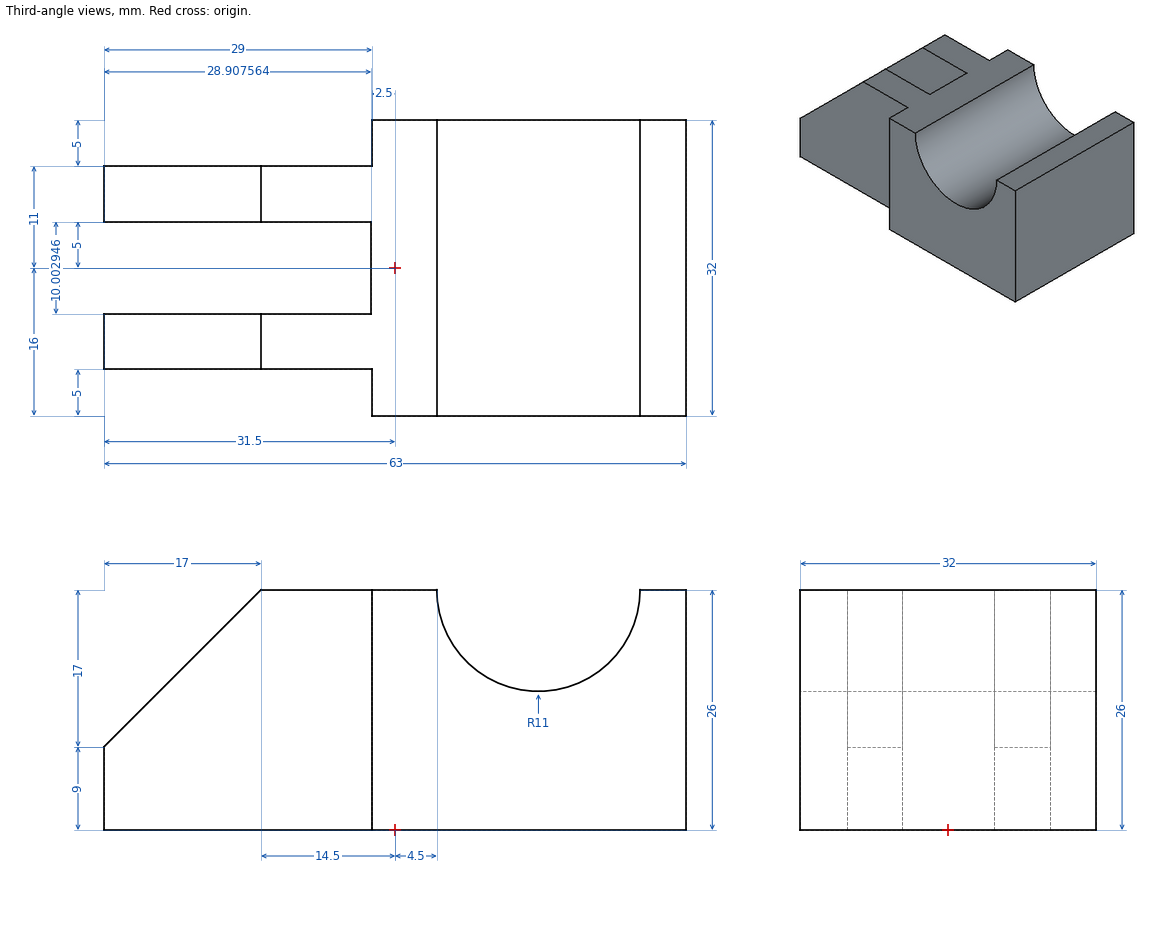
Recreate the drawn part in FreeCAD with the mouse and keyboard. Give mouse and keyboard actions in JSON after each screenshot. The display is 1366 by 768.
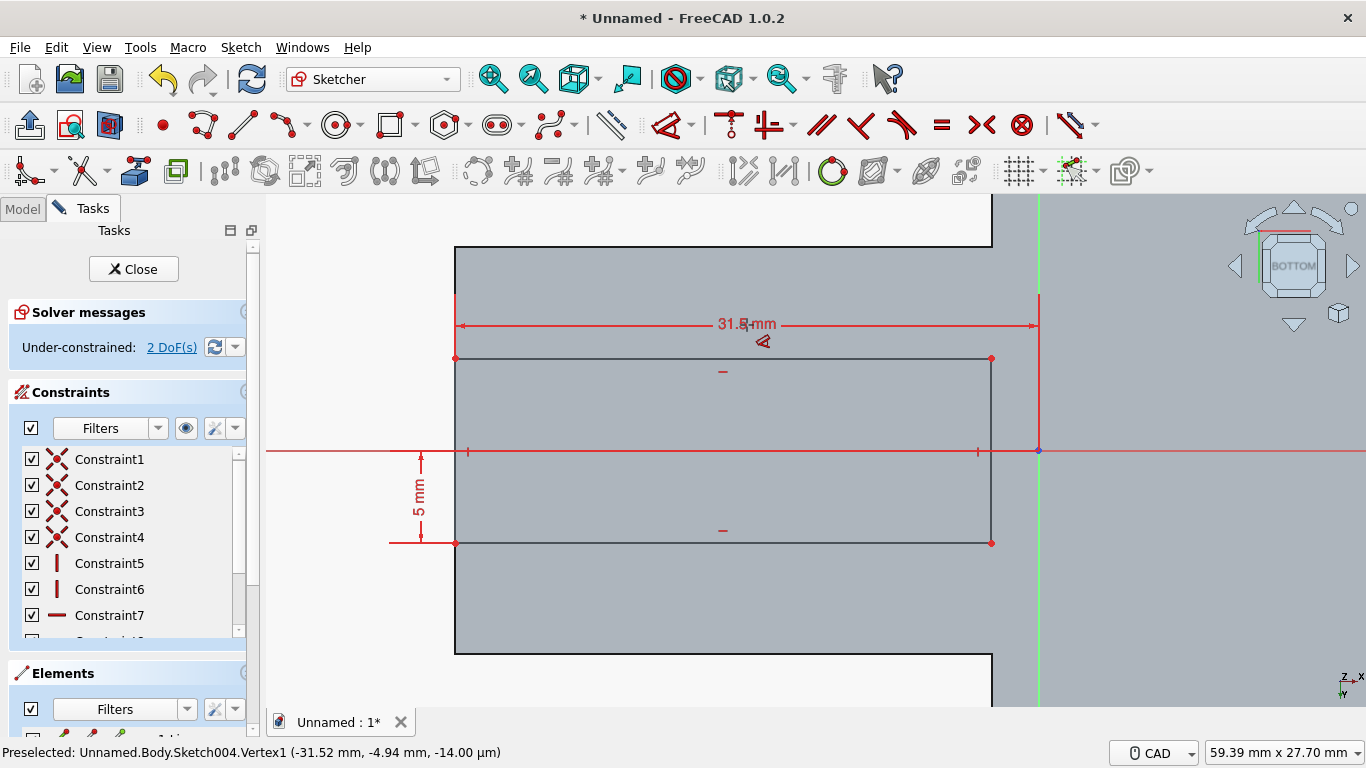
{"action": "left_click", "coordinate": [455, 414]}
{"action": "left_click", "coordinate": [421, 409]}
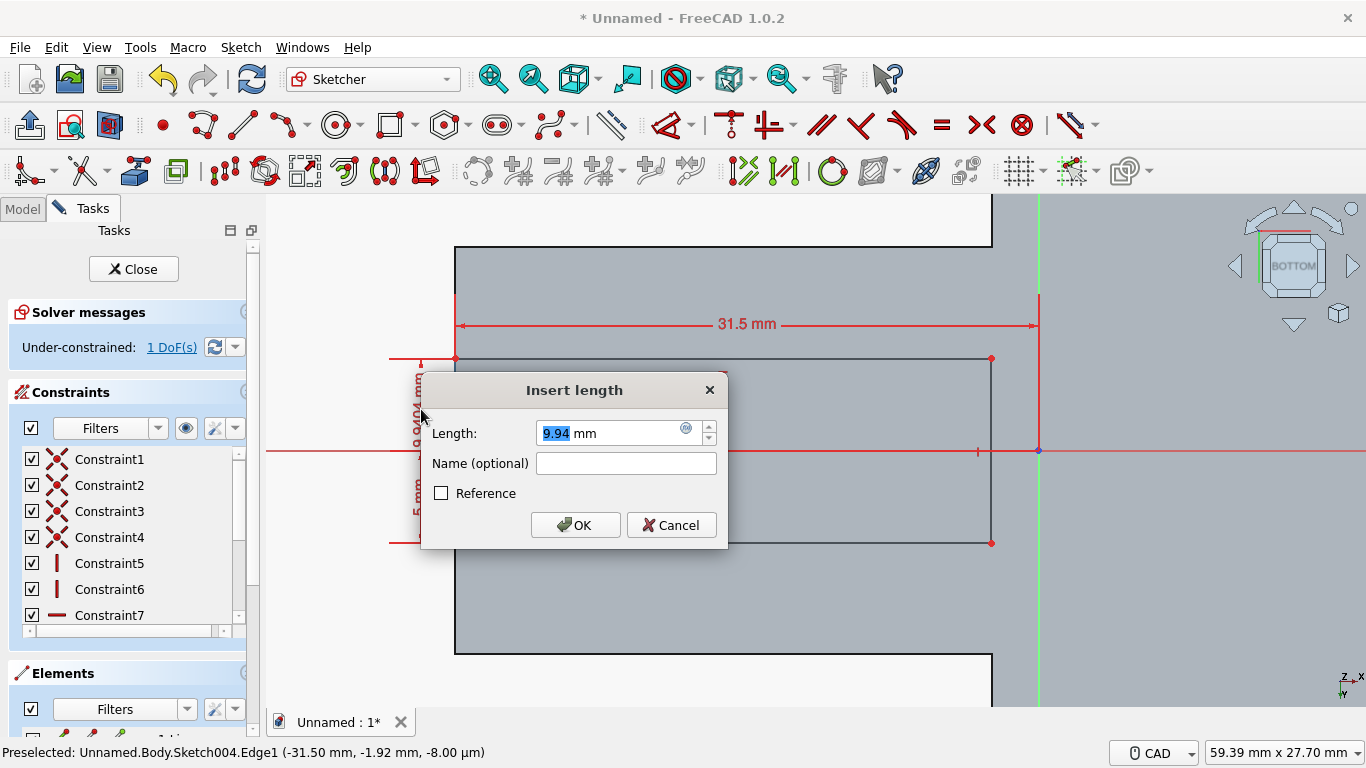
{"action": "type", "text": "10.002946"}
{"action": "key", "text": "Return"}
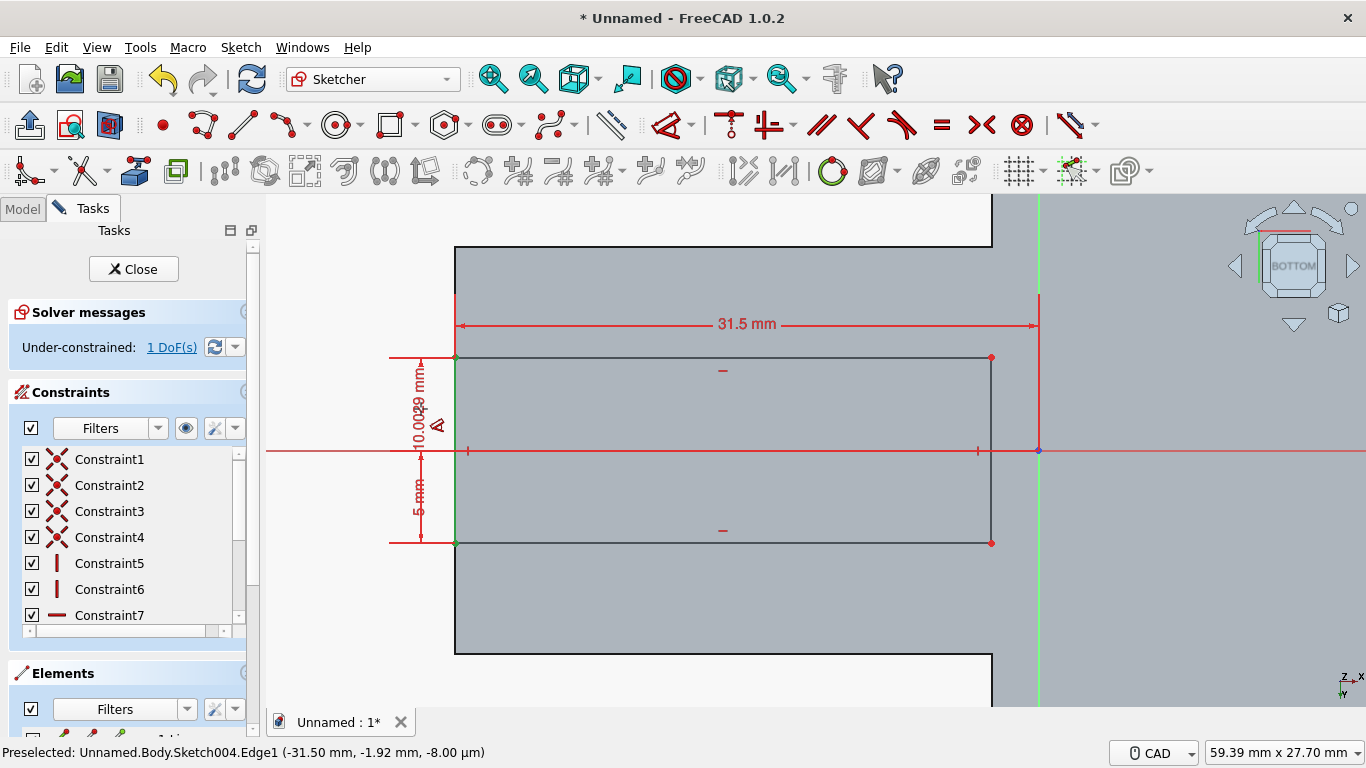
{"action": "left_click", "coordinate": [616, 543]}
{"action": "left_click", "coordinate": [723, 577]}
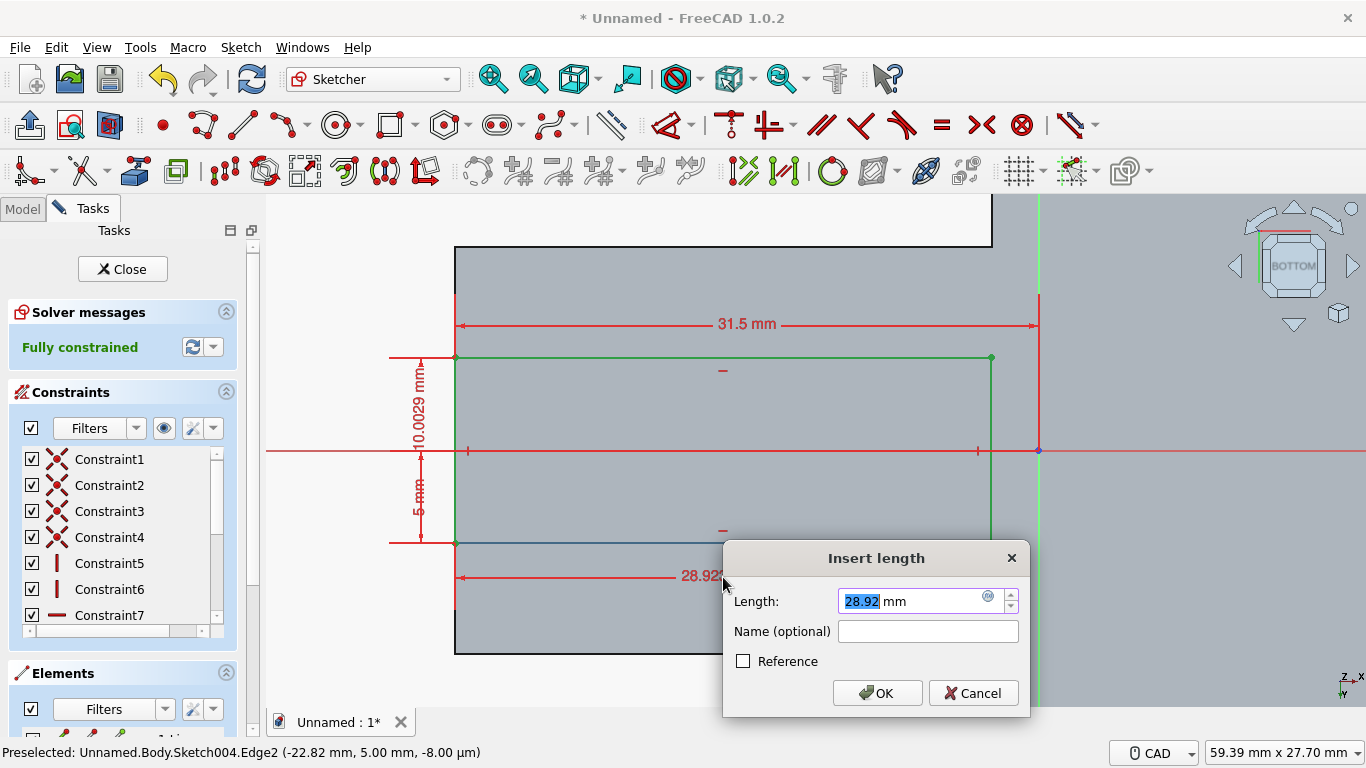
{"action": "type", "text": "28.907564"}
{"action": "key", "text": "Return"}
{"action": "key", "text": "Escape"}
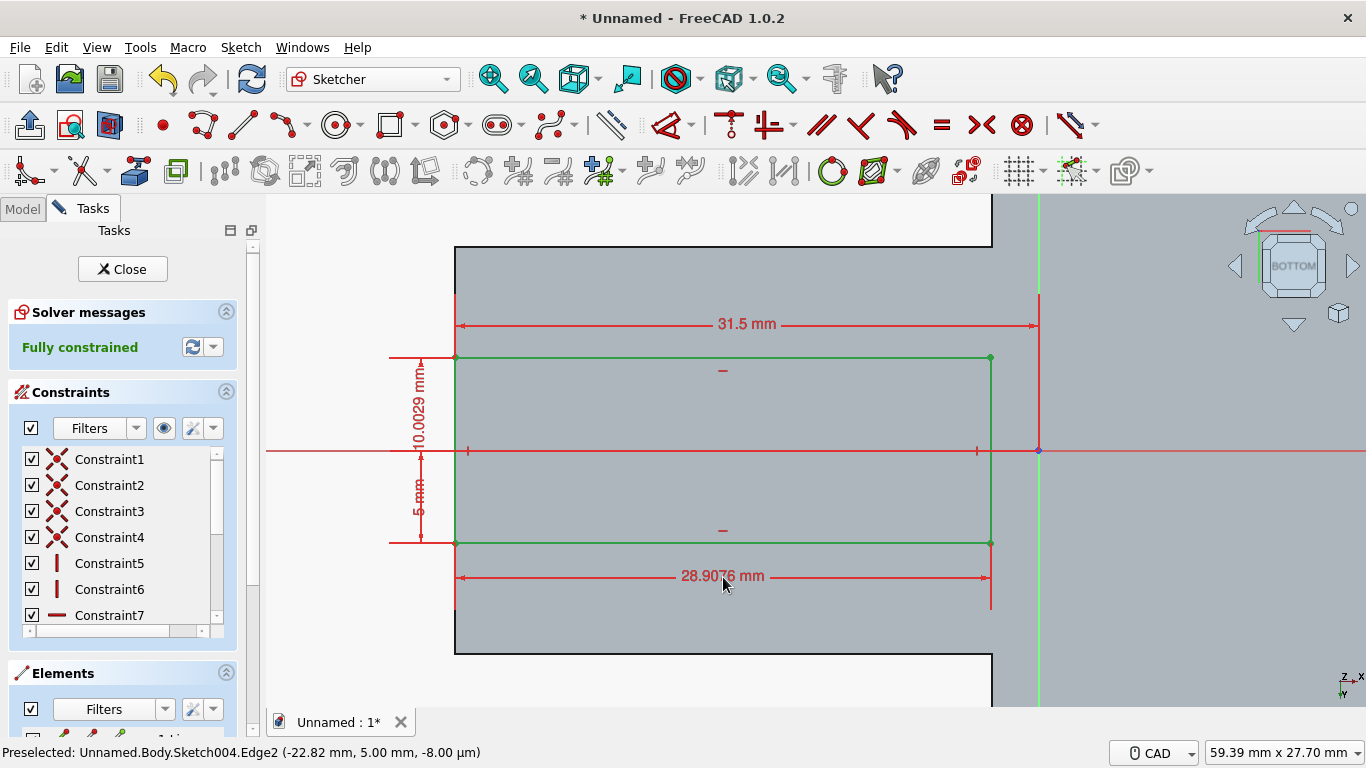
{"action": "left_click", "coordinate": [123, 269]}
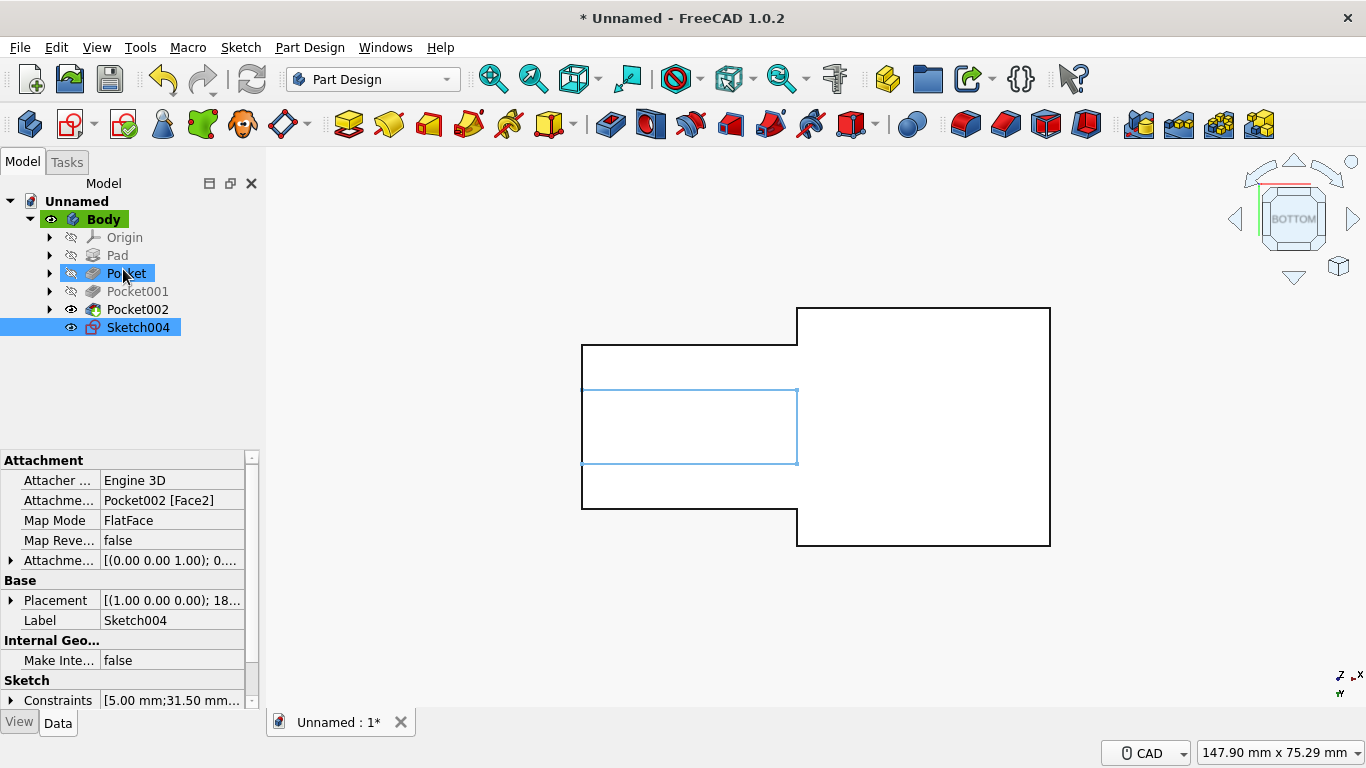
{"action": "left_click", "coordinate": [612, 124]}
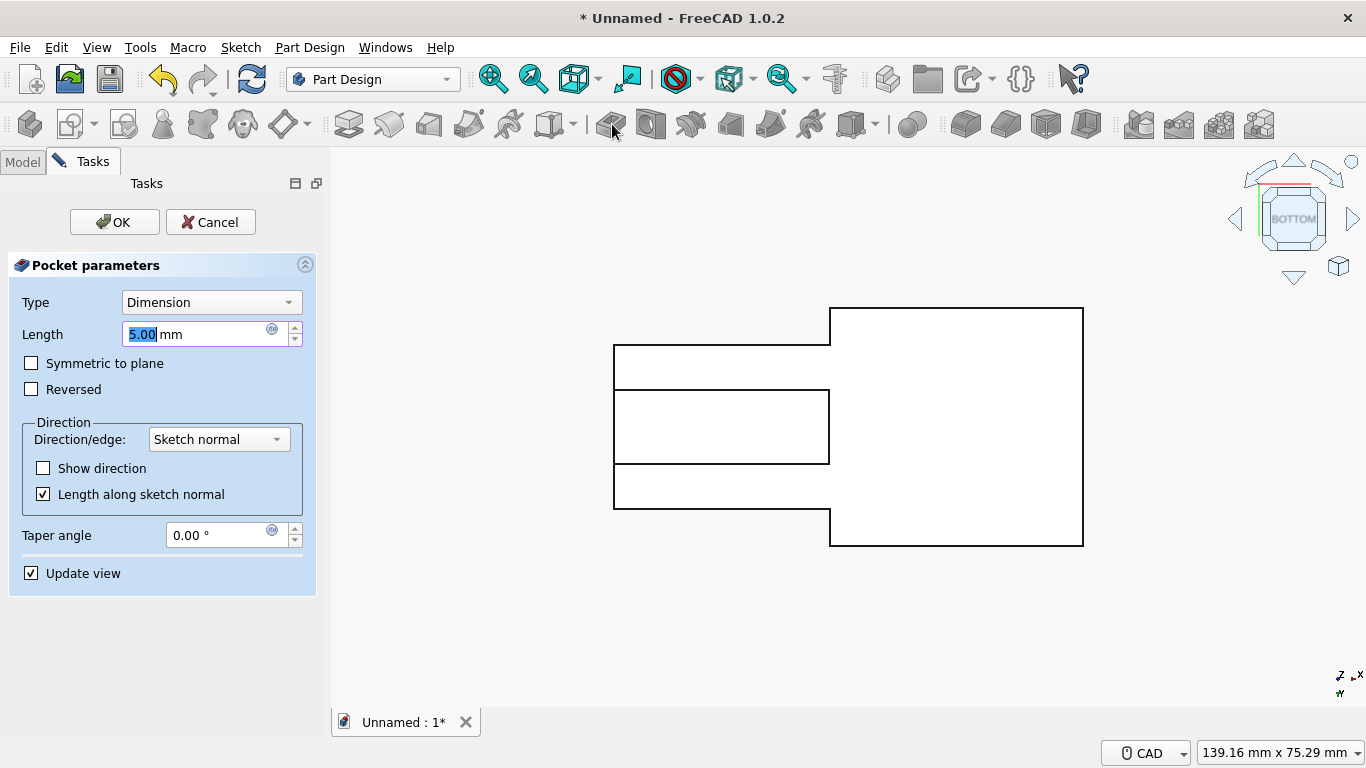
{"action": "left_click", "coordinate": [212, 302]}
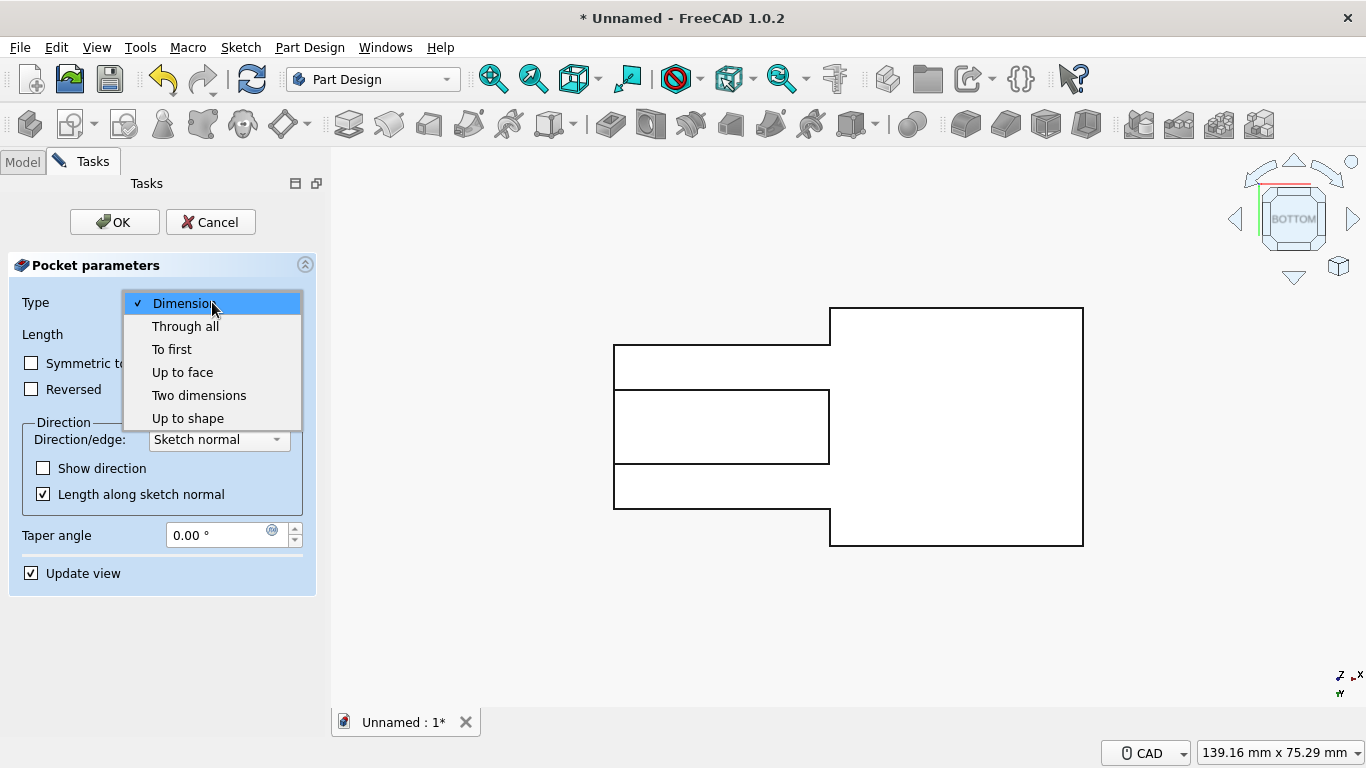
{"action": "left_click", "coordinate": [212, 326]}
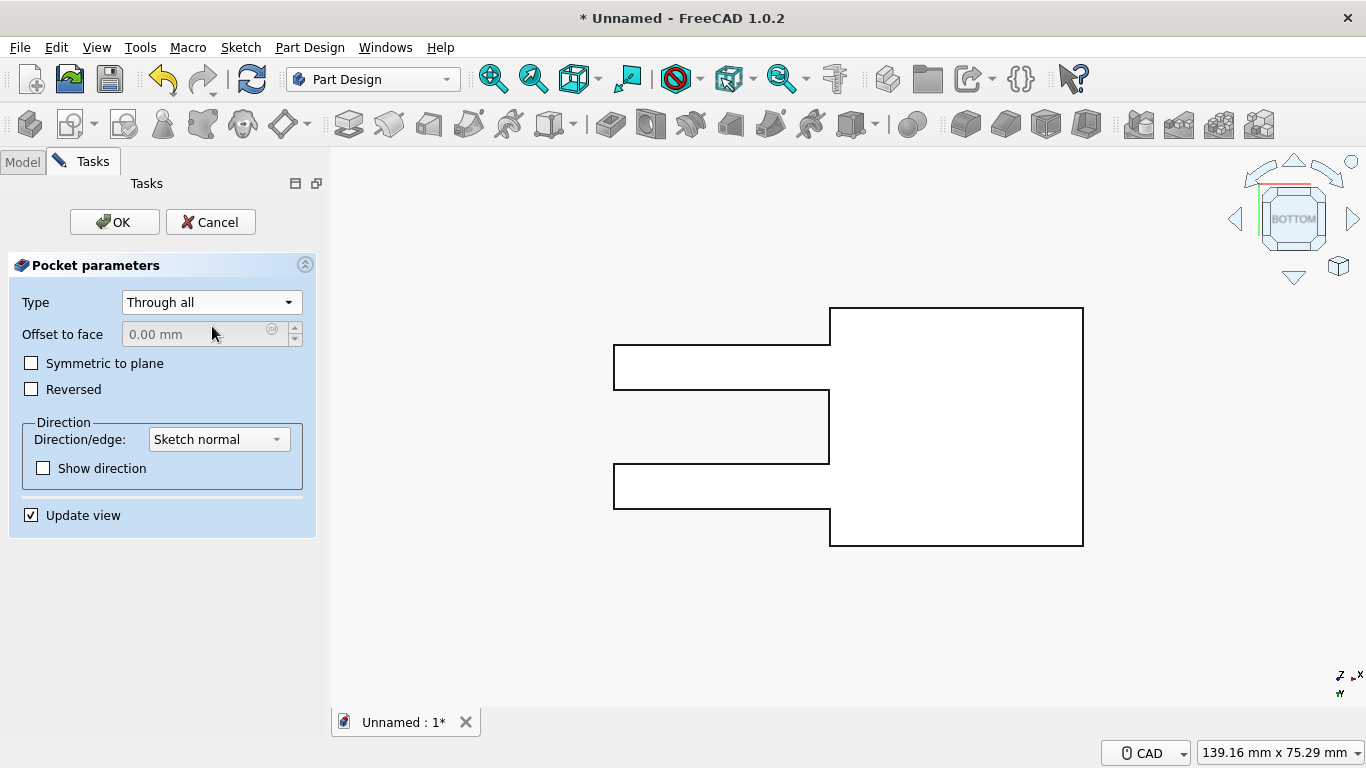
{"action": "left_click", "coordinate": [115, 222]}